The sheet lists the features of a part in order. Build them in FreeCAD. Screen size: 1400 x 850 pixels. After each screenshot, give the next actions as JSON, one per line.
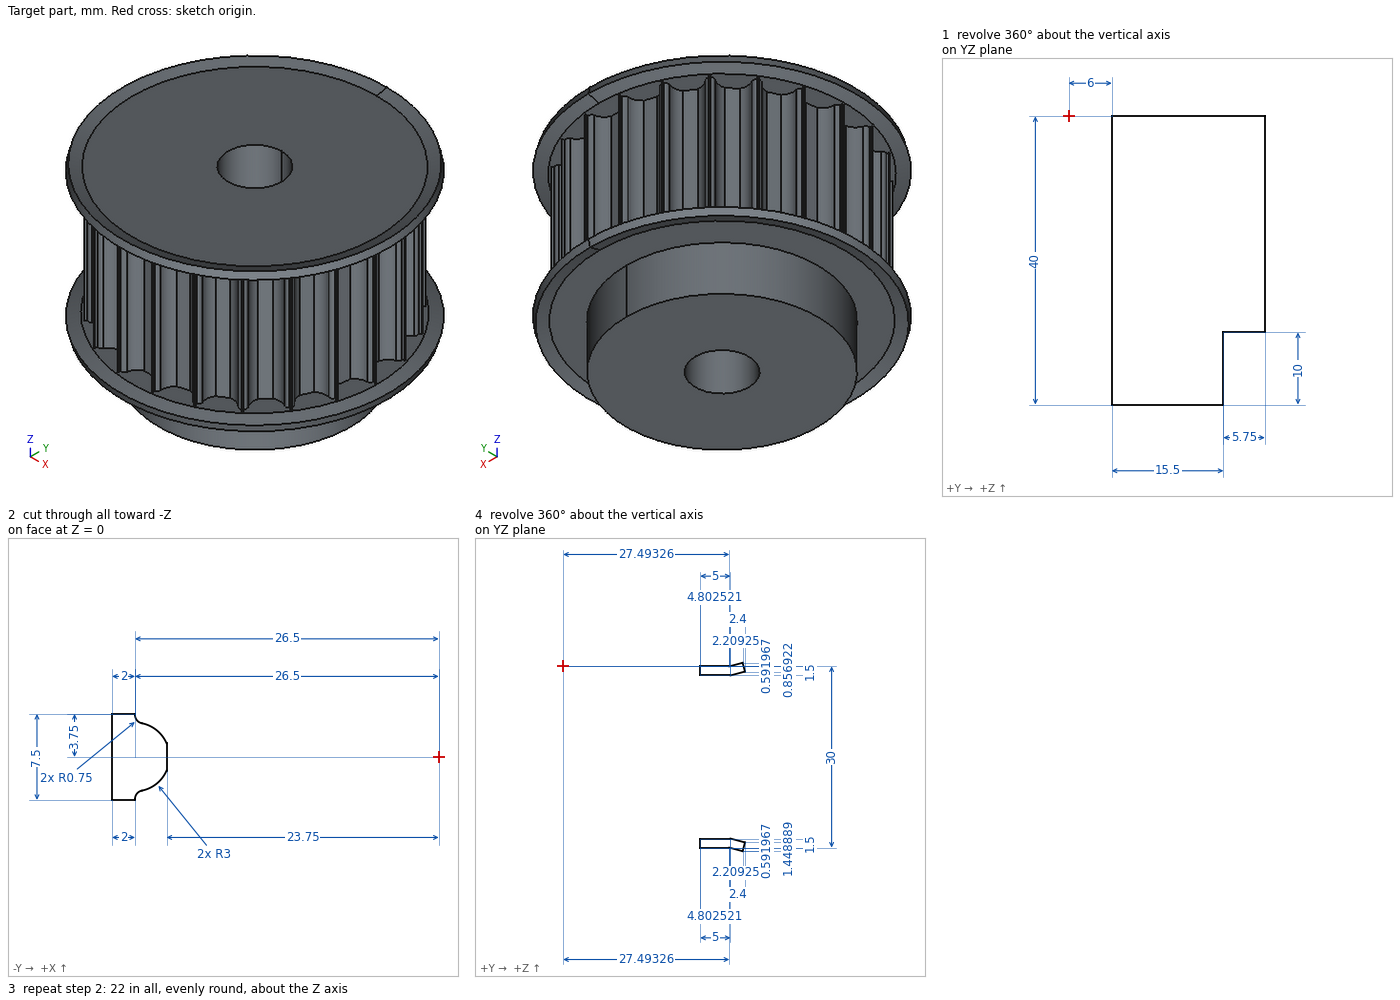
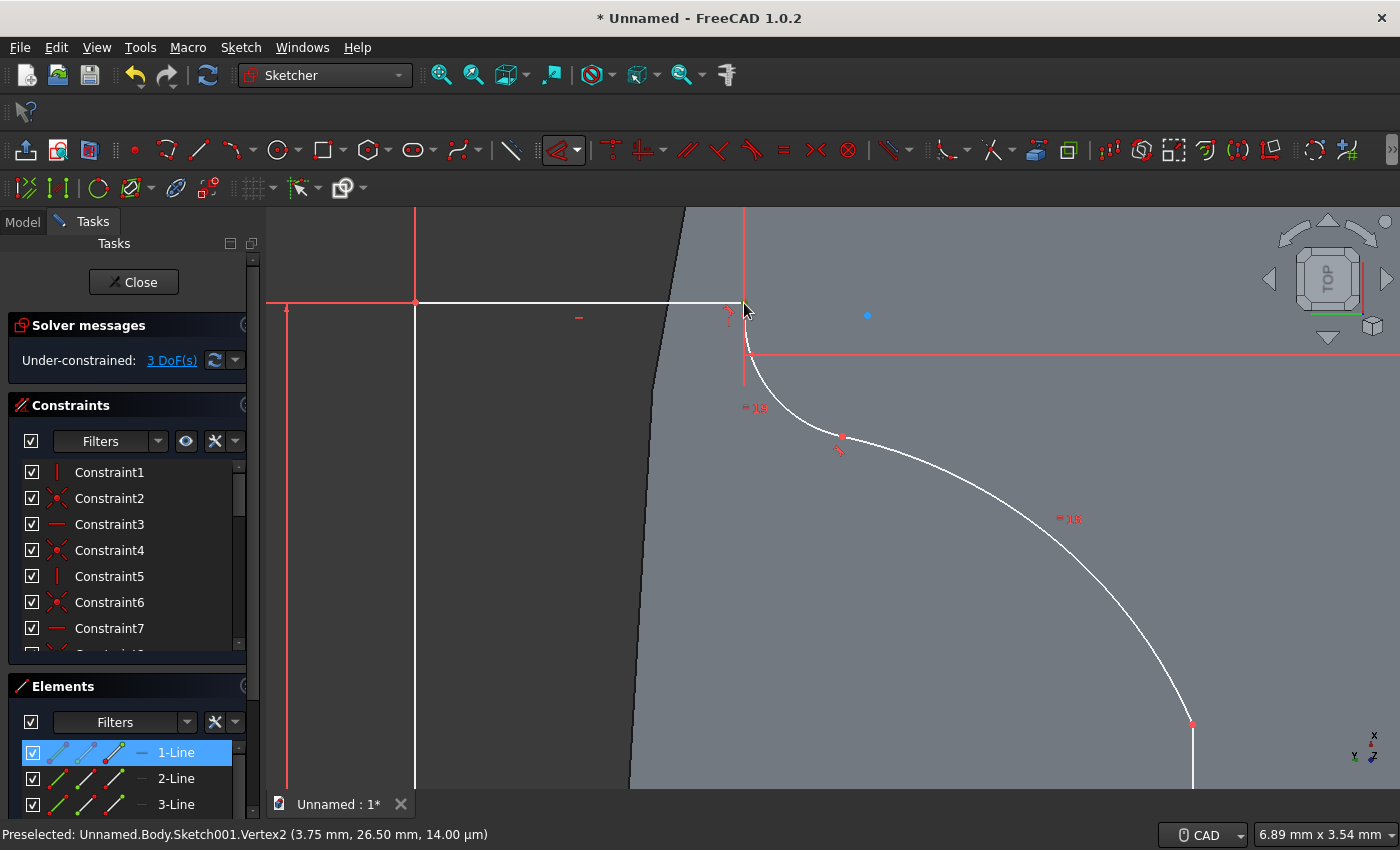
{"action": "left_click", "coordinate": [580, 150]}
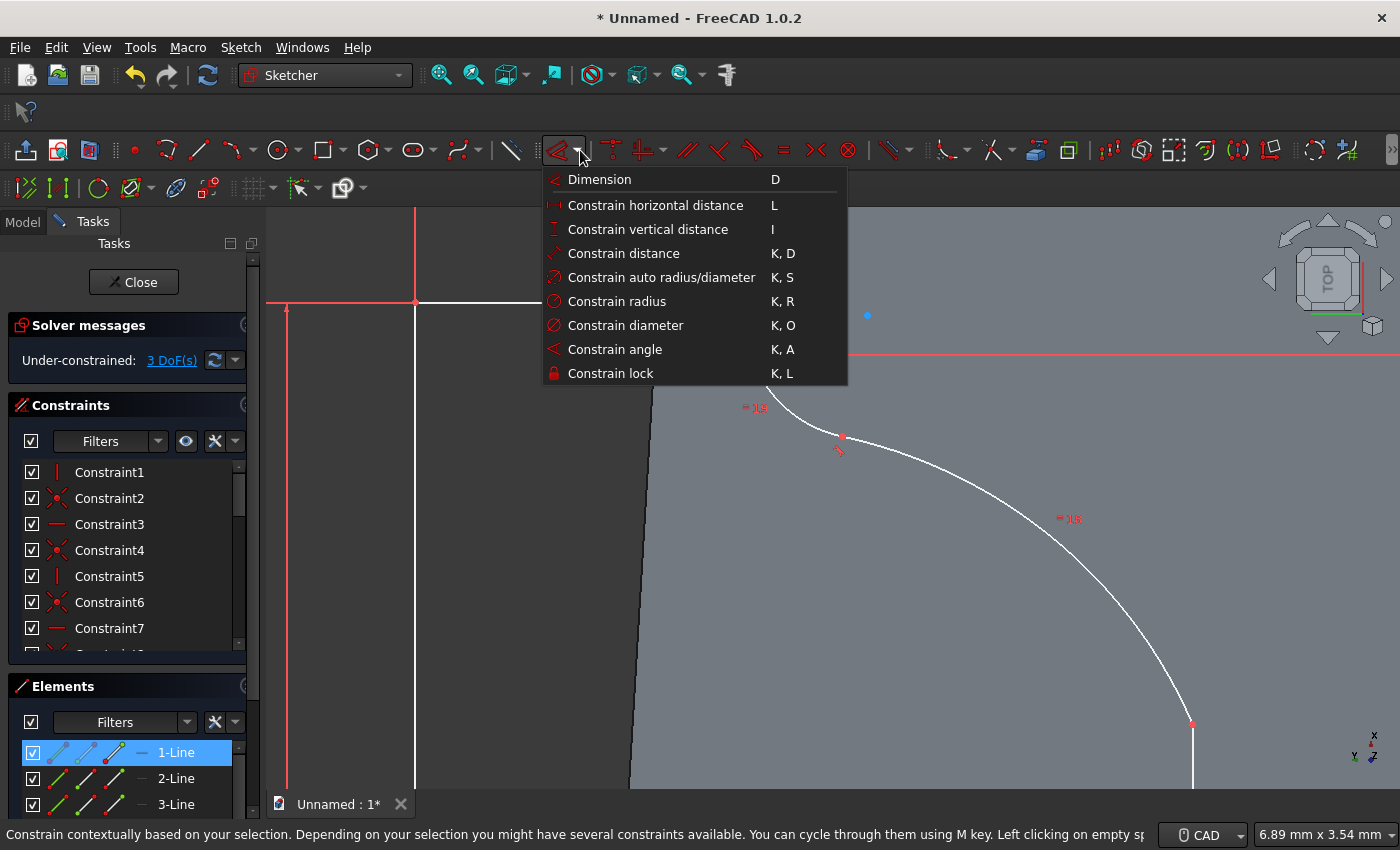
{"action": "left_click", "coordinate": [695, 229]}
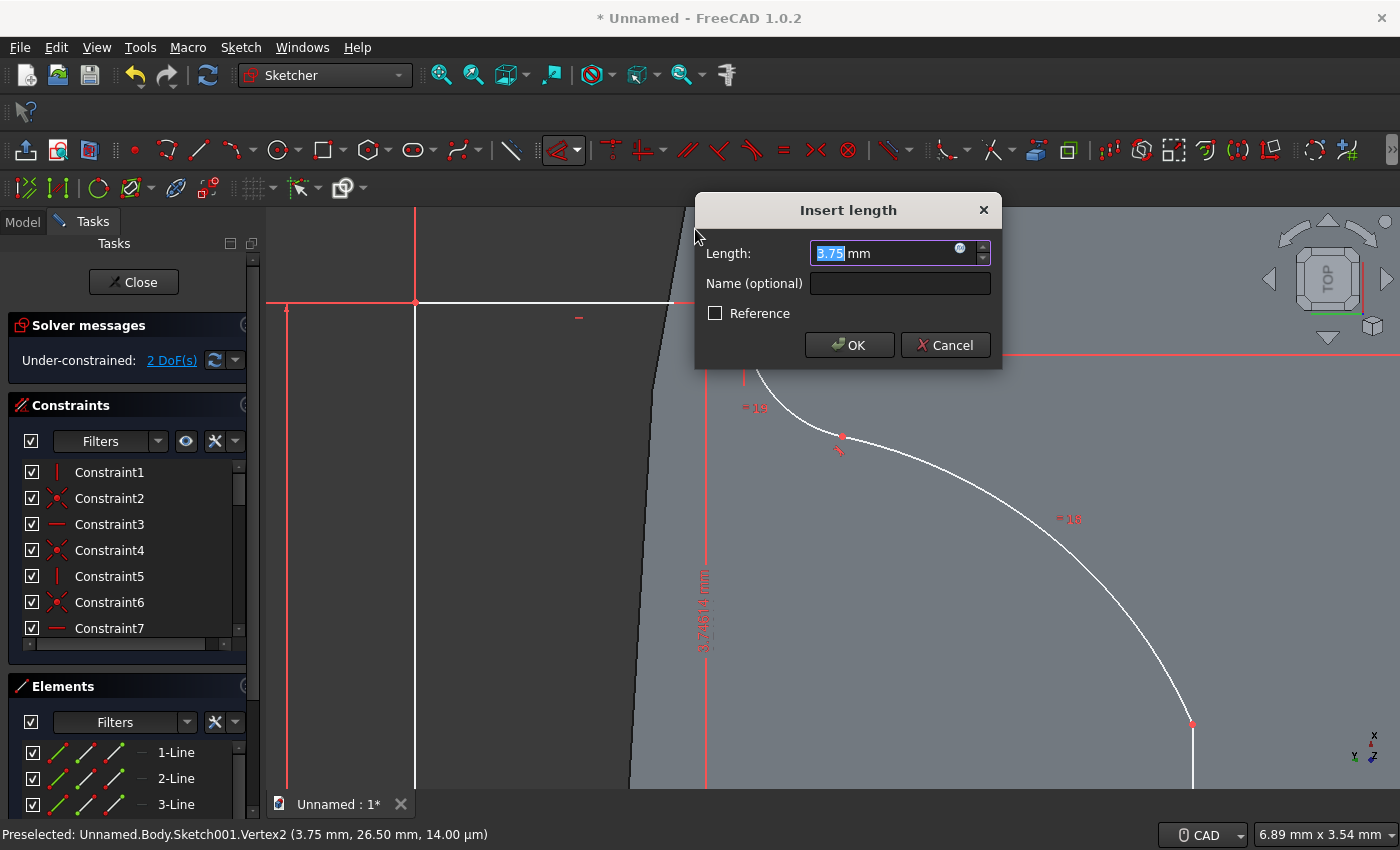
{"action": "type", "text": "3.75"}
{"action": "key", "text": "Return"}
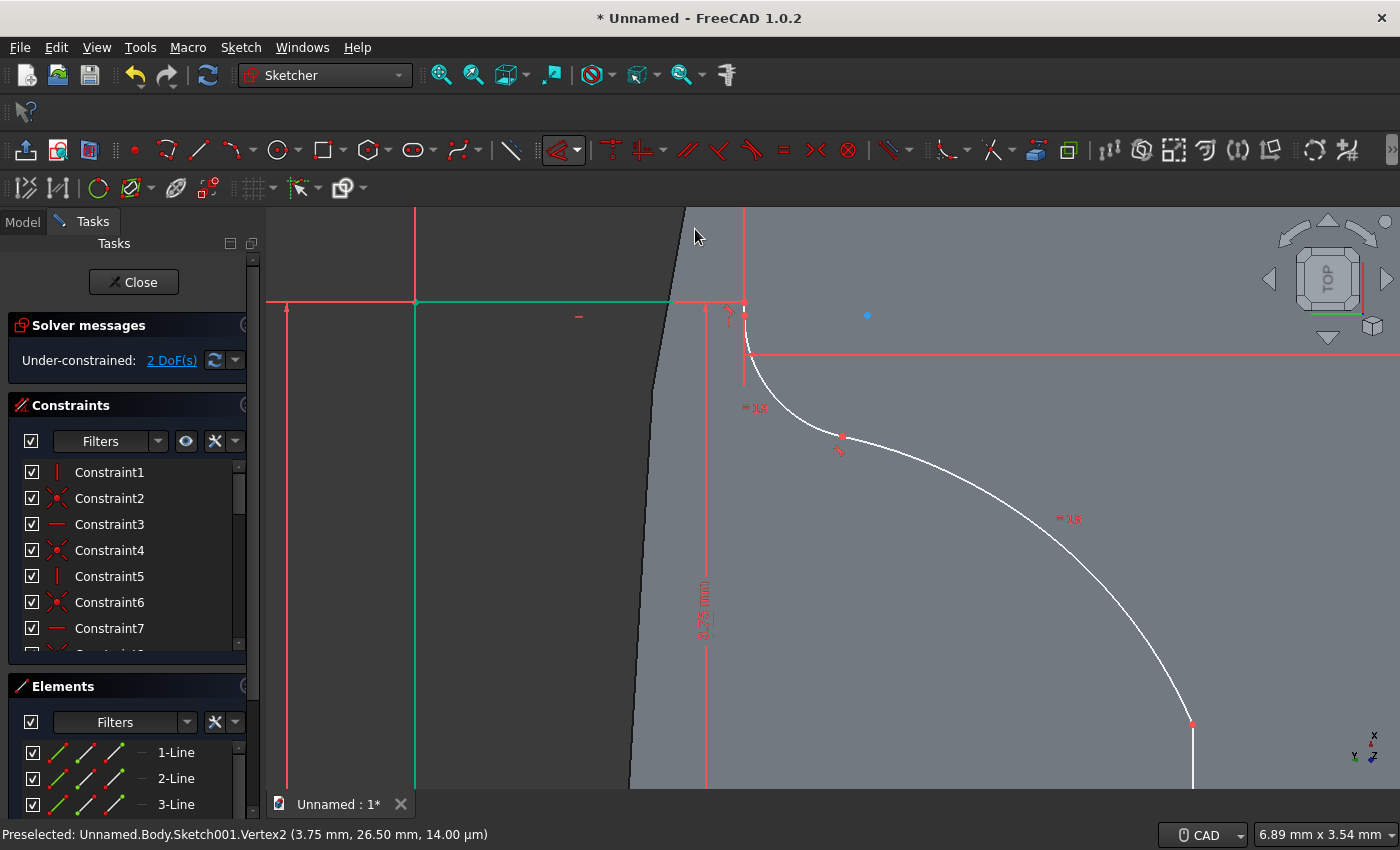
{"action": "scroll", "coordinate": [747, 316], "scroll_direction": "down", "scroll_amount": 6}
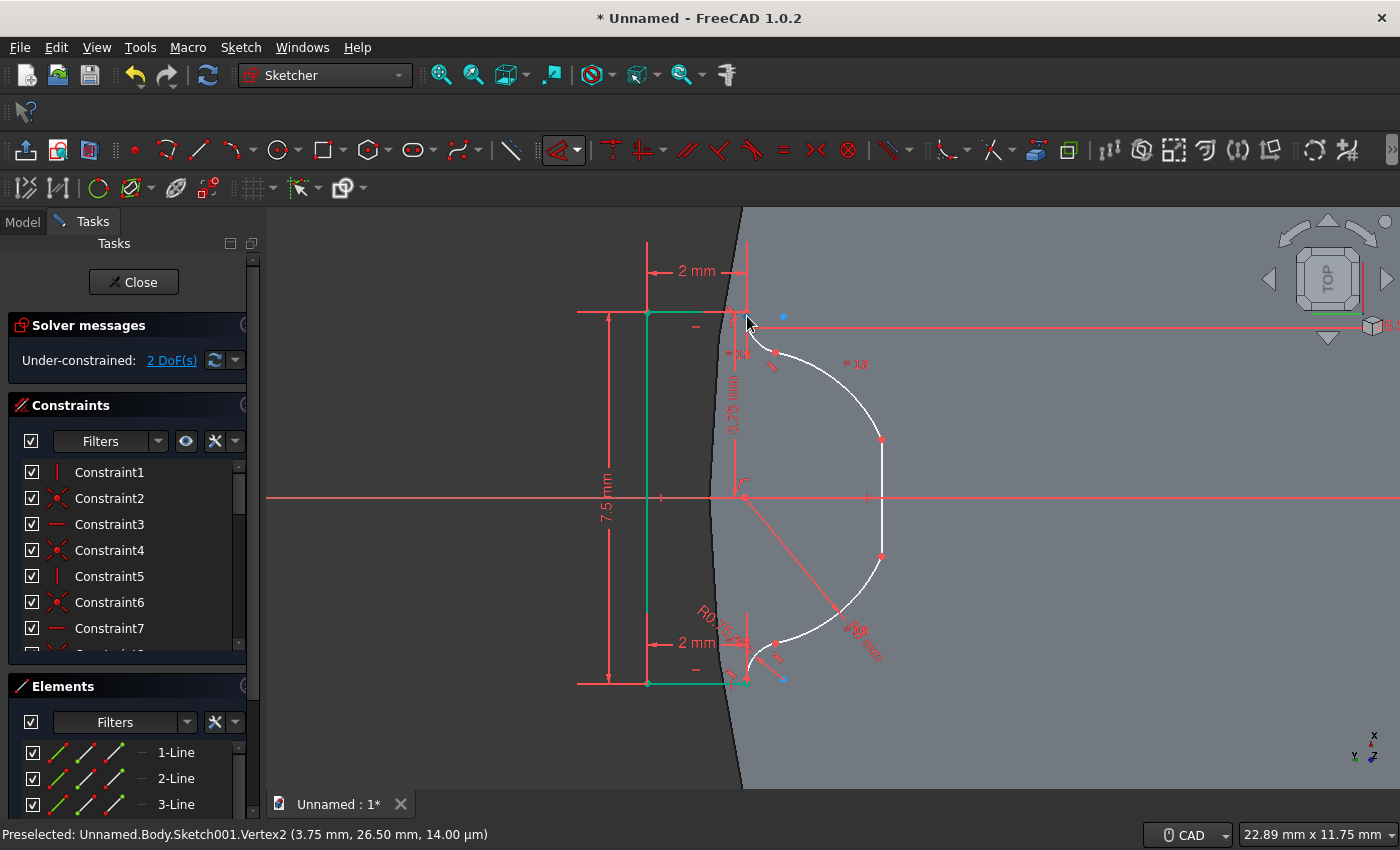
{"action": "left_click", "coordinate": [745, 498]}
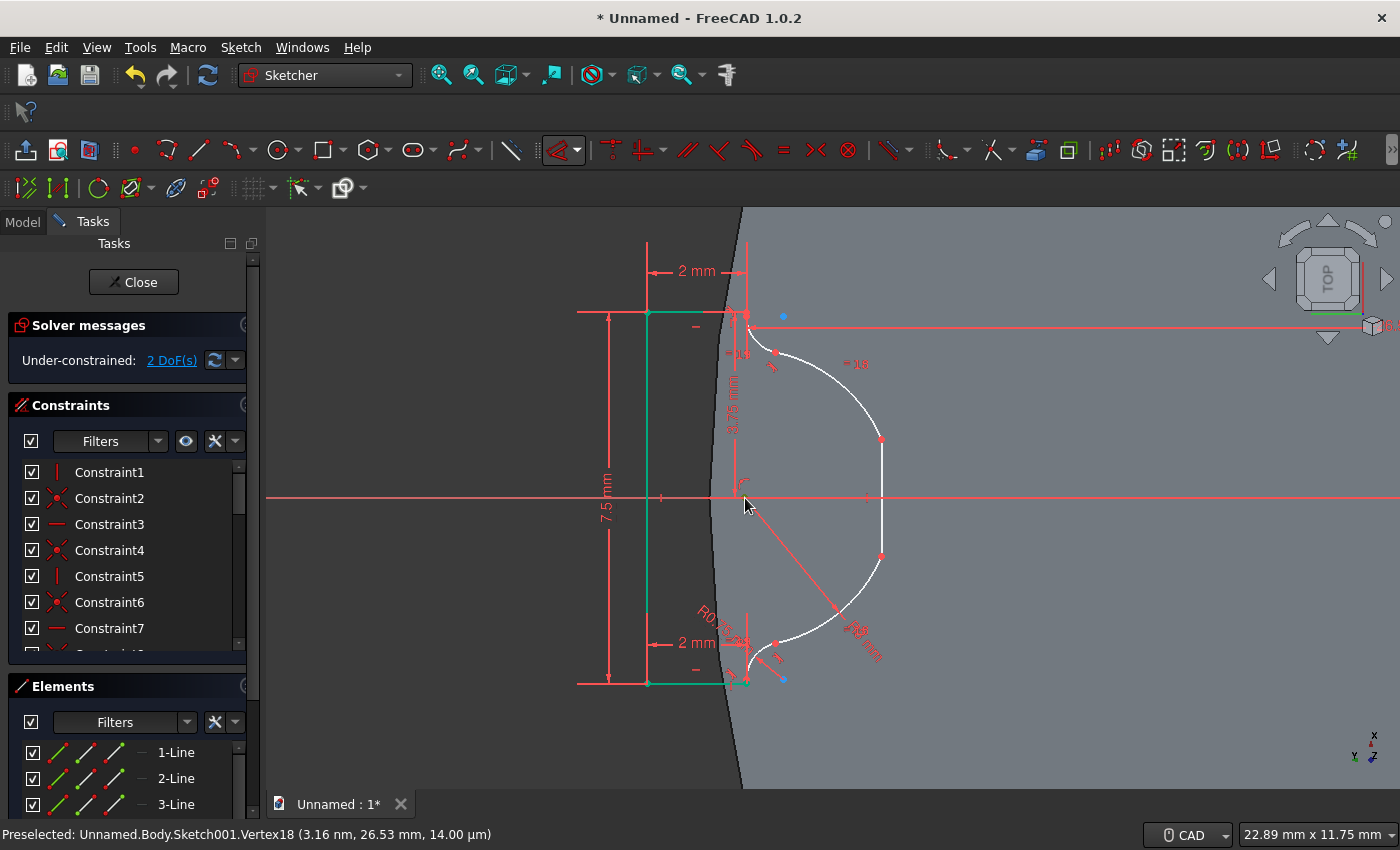
{"action": "key", "text": "l"}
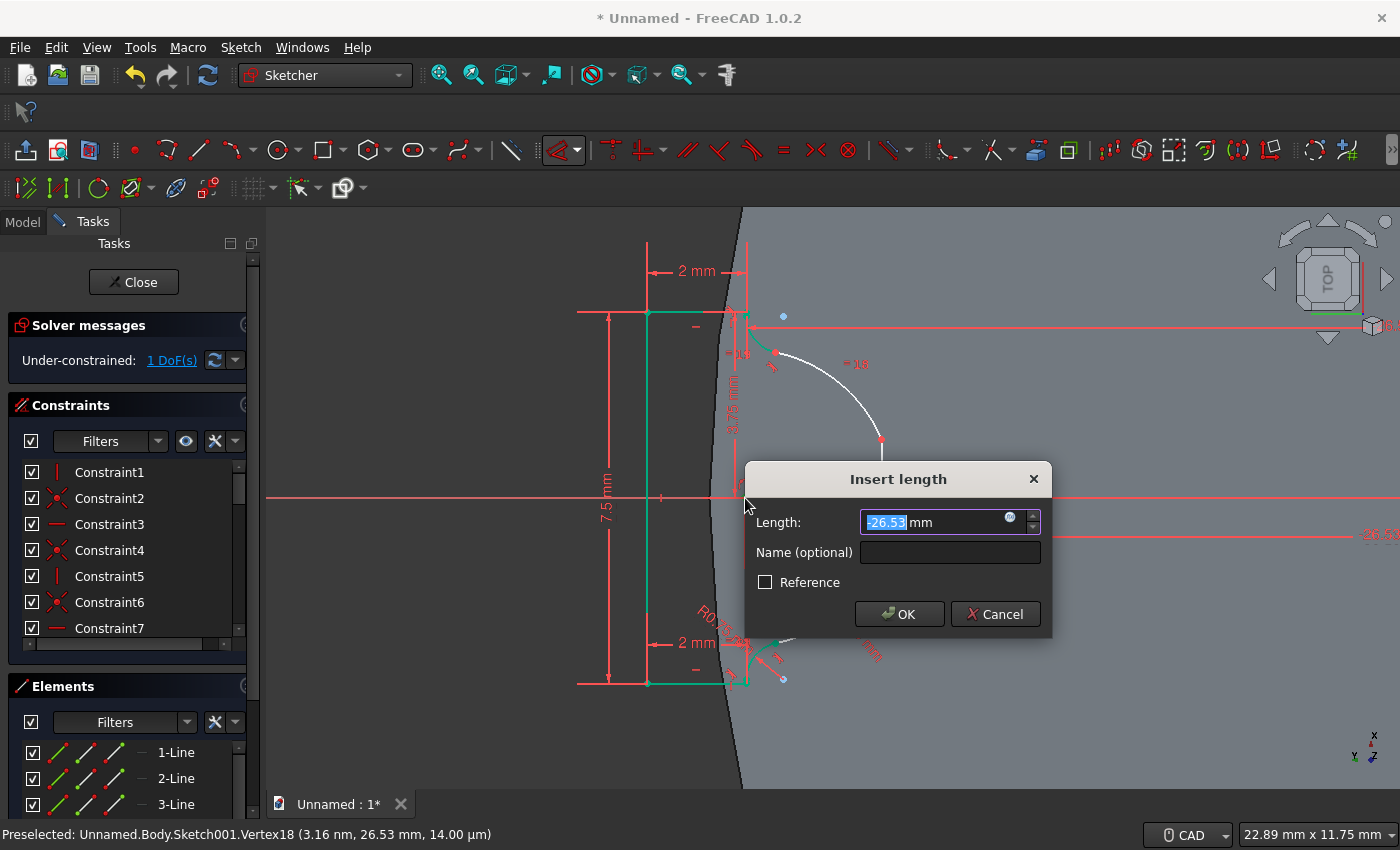
{"action": "type", "text": "-26.5"}
{"action": "key", "text": "Return"}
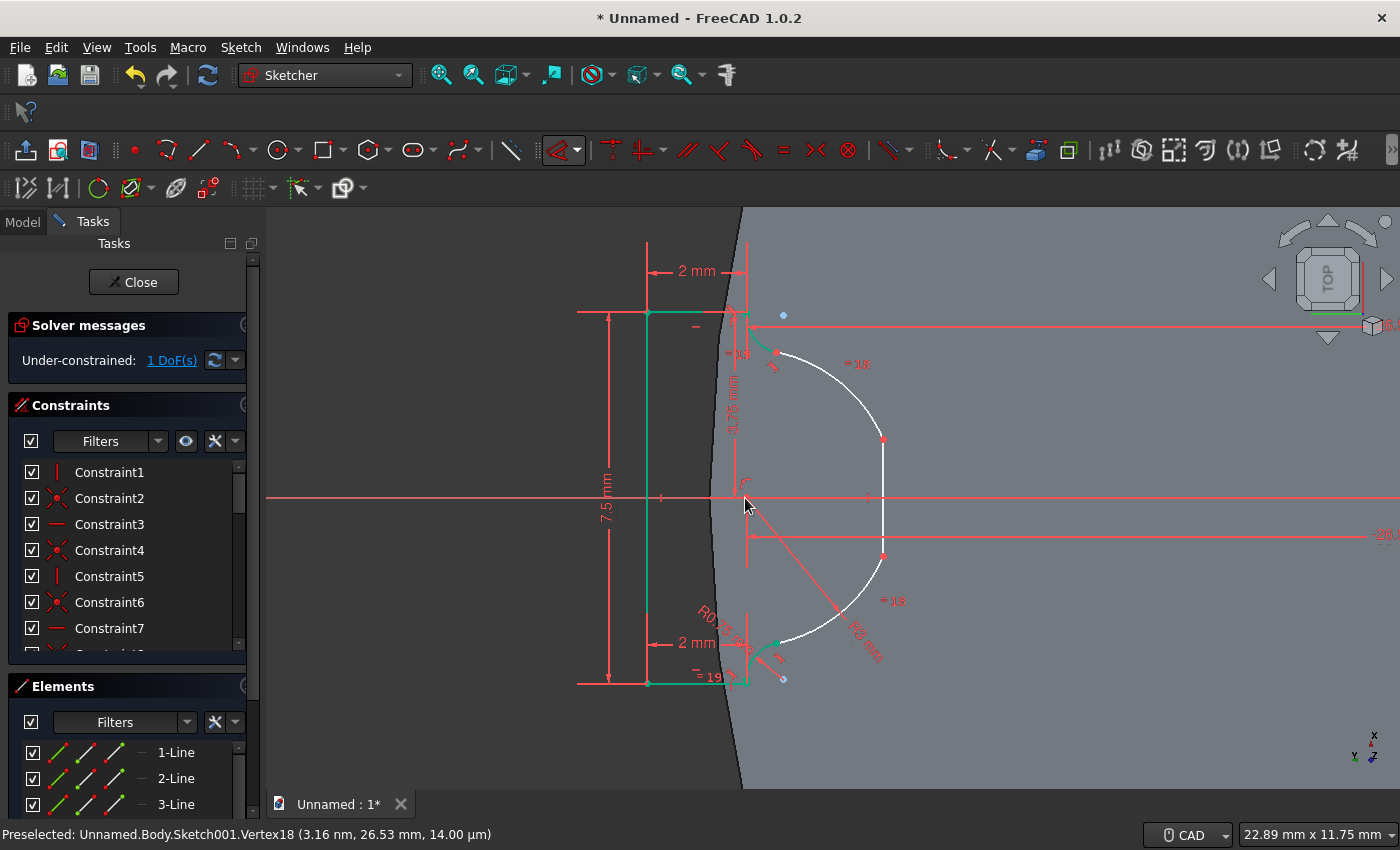
{"action": "left_click", "coordinate": [883, 556]}